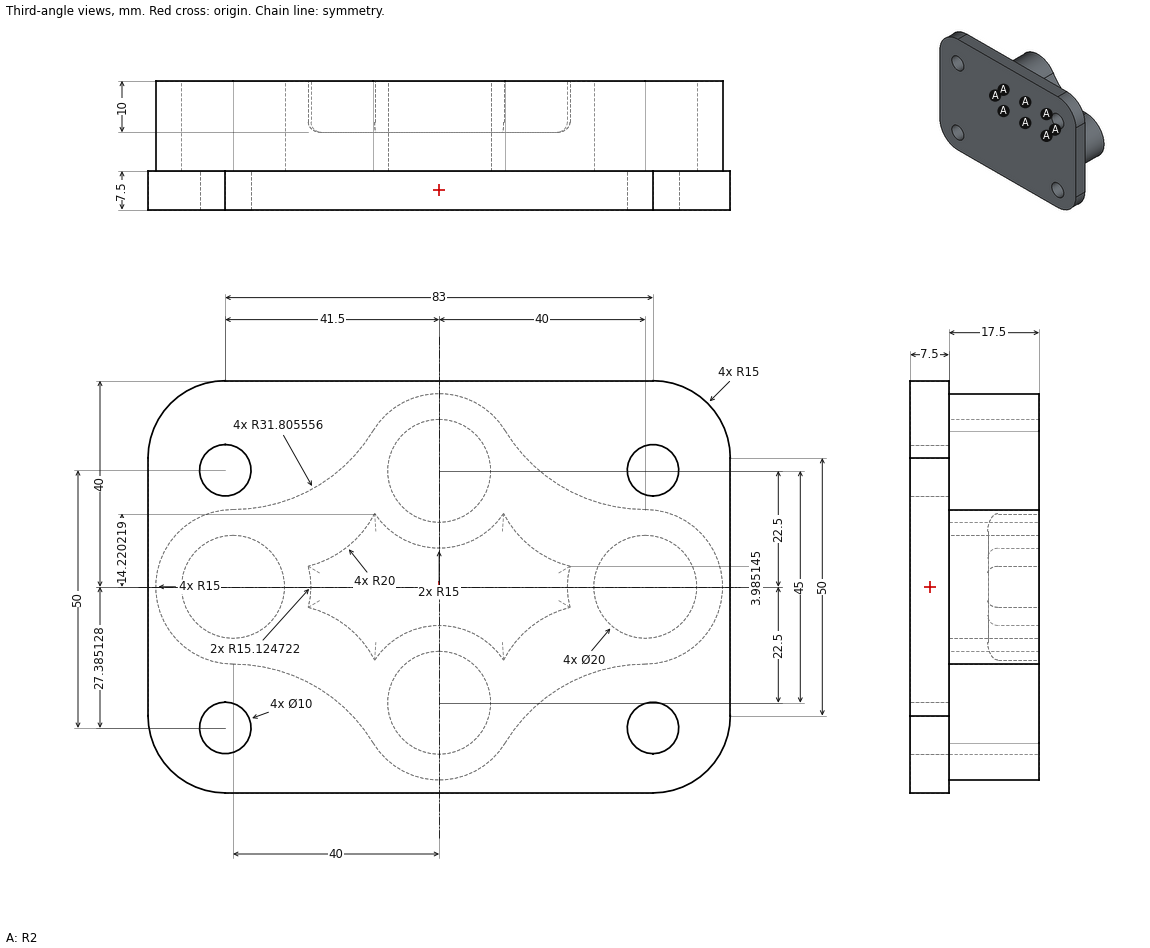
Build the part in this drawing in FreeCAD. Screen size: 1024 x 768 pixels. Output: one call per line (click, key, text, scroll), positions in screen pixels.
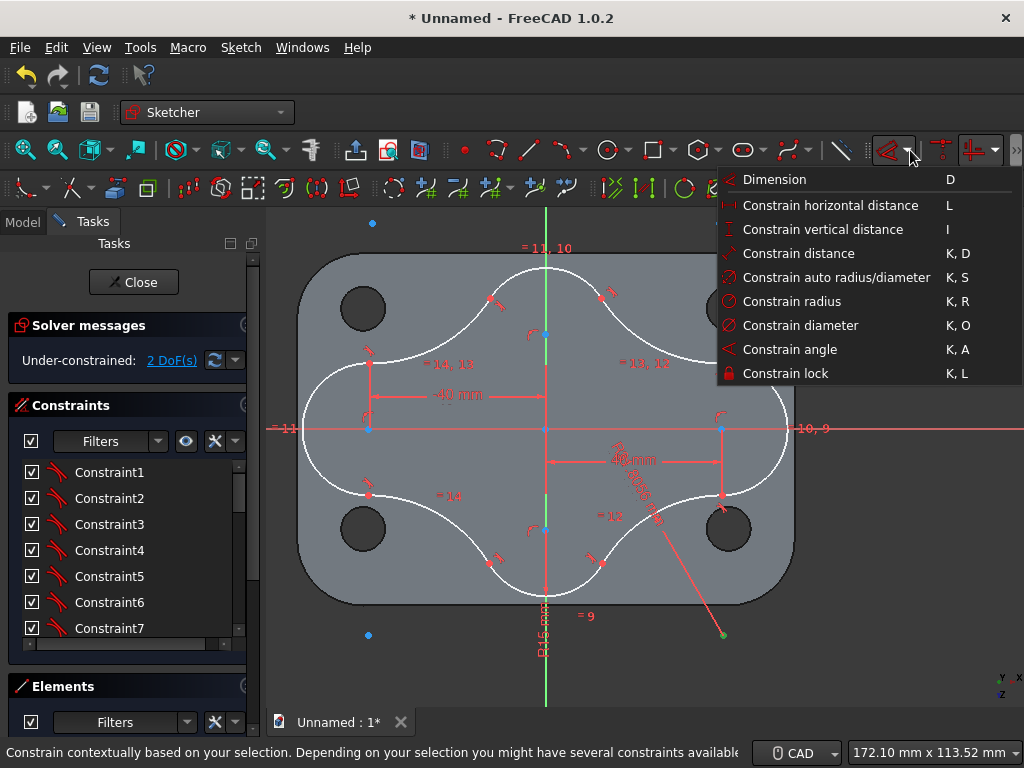
click(870, 205)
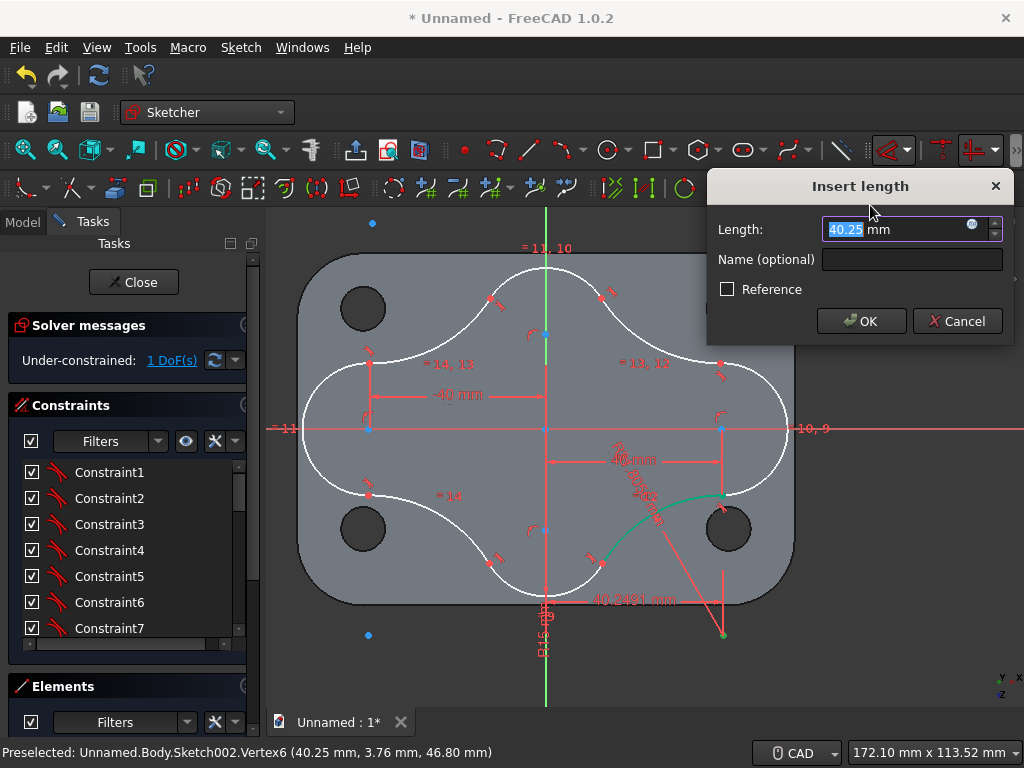
text(40)
key(Return)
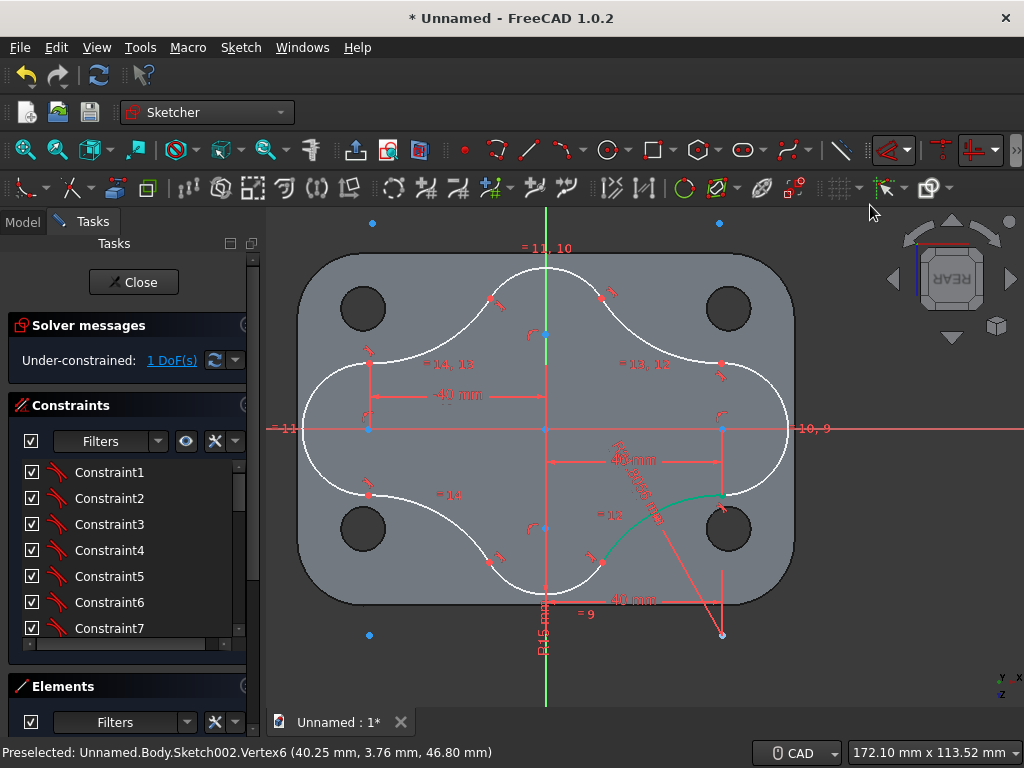
scroll(715, 582, down, 1)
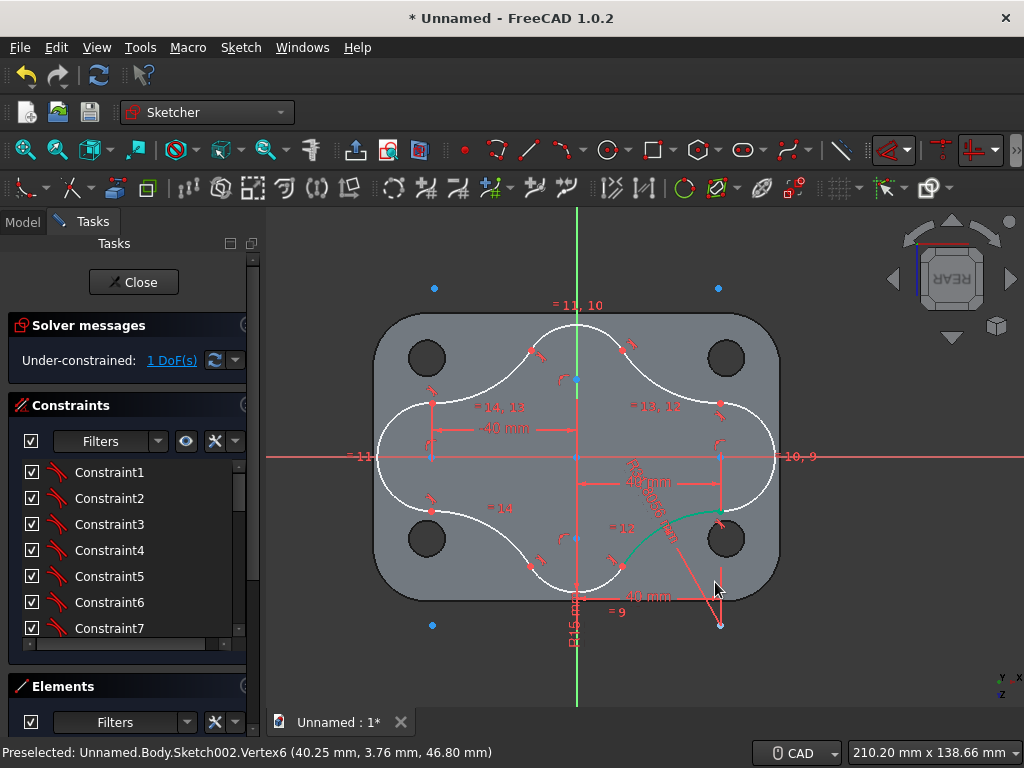
click(719, 288)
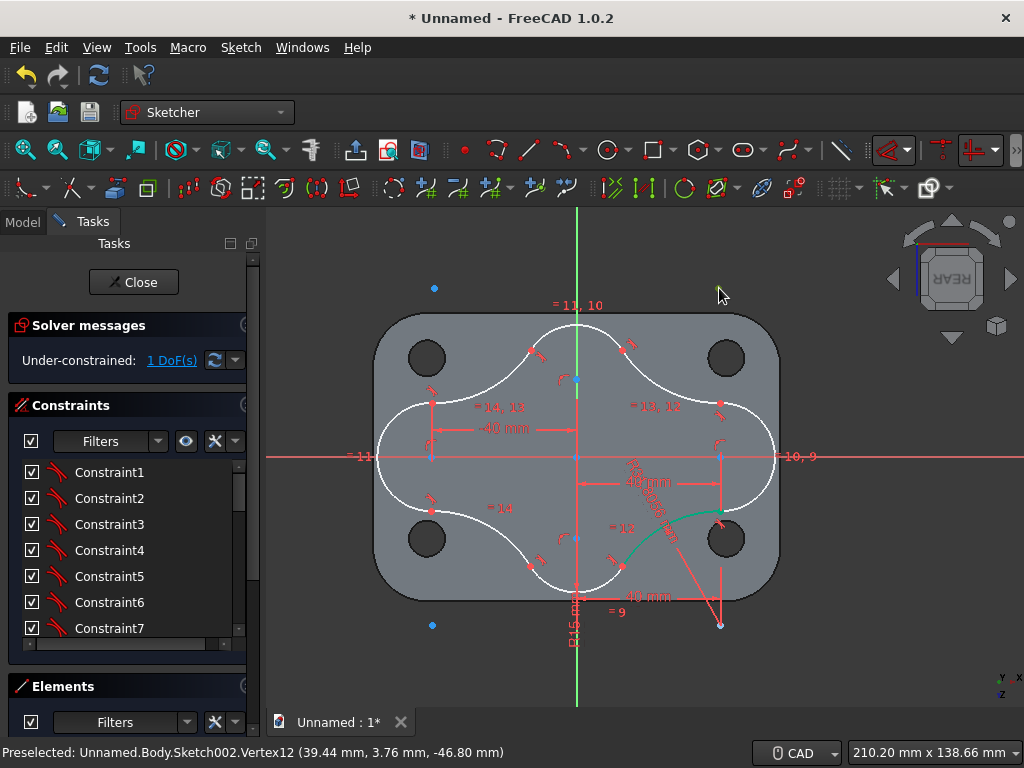
click(910, 150)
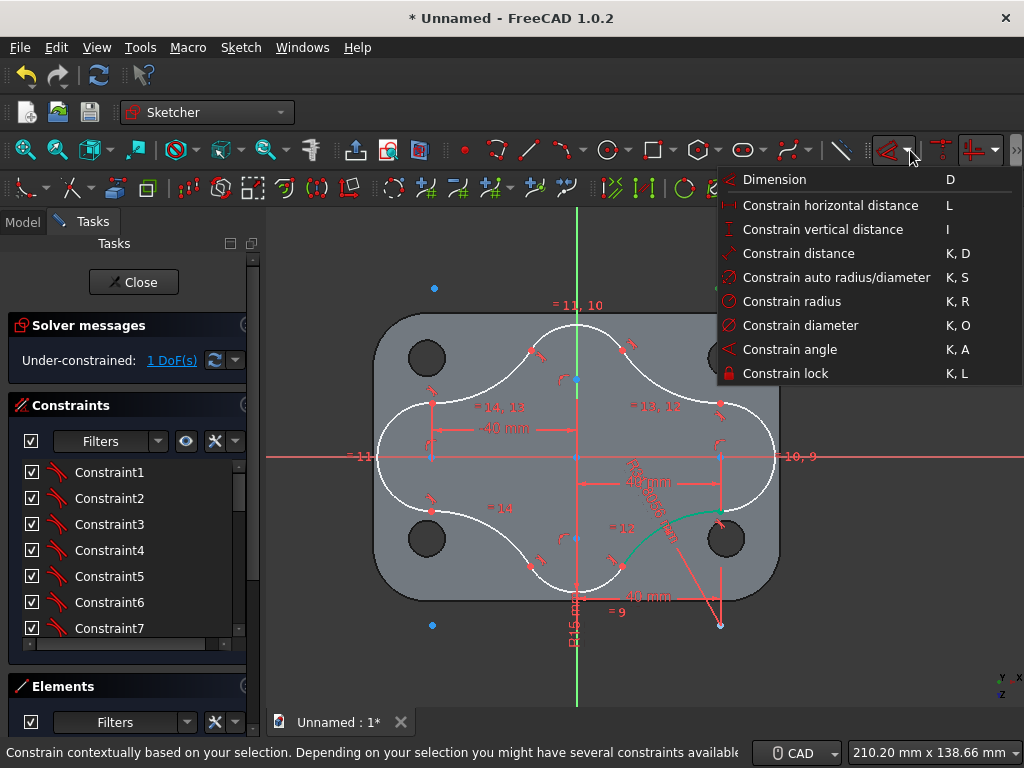
click(870, 205)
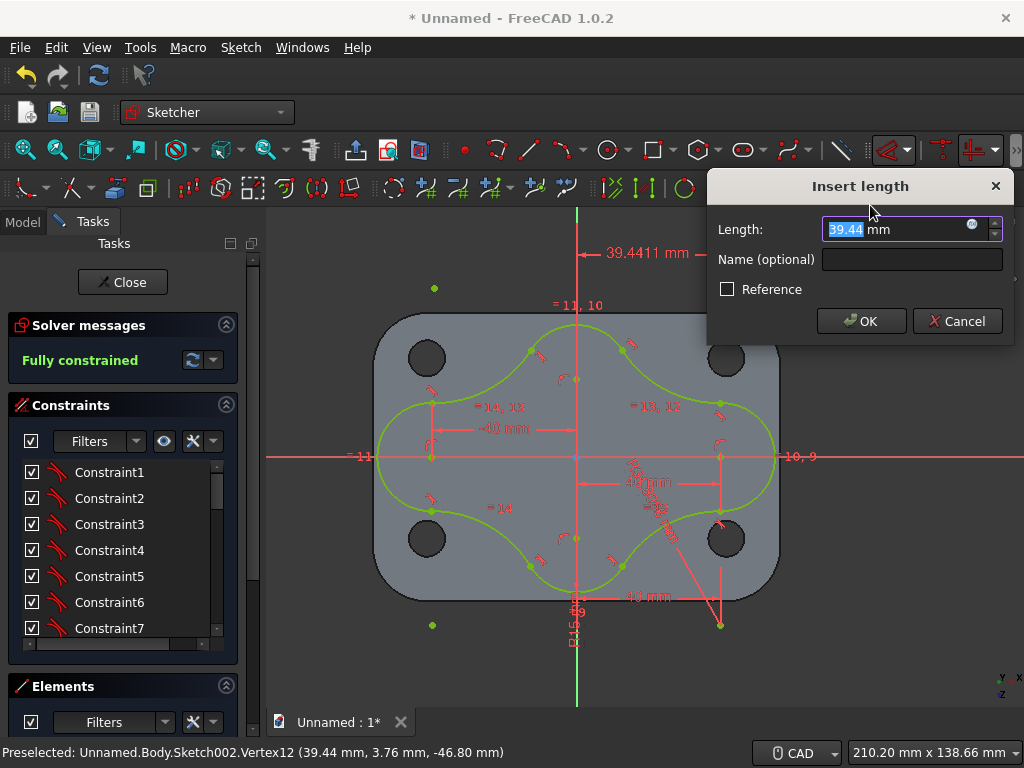
text(40)
key(Return)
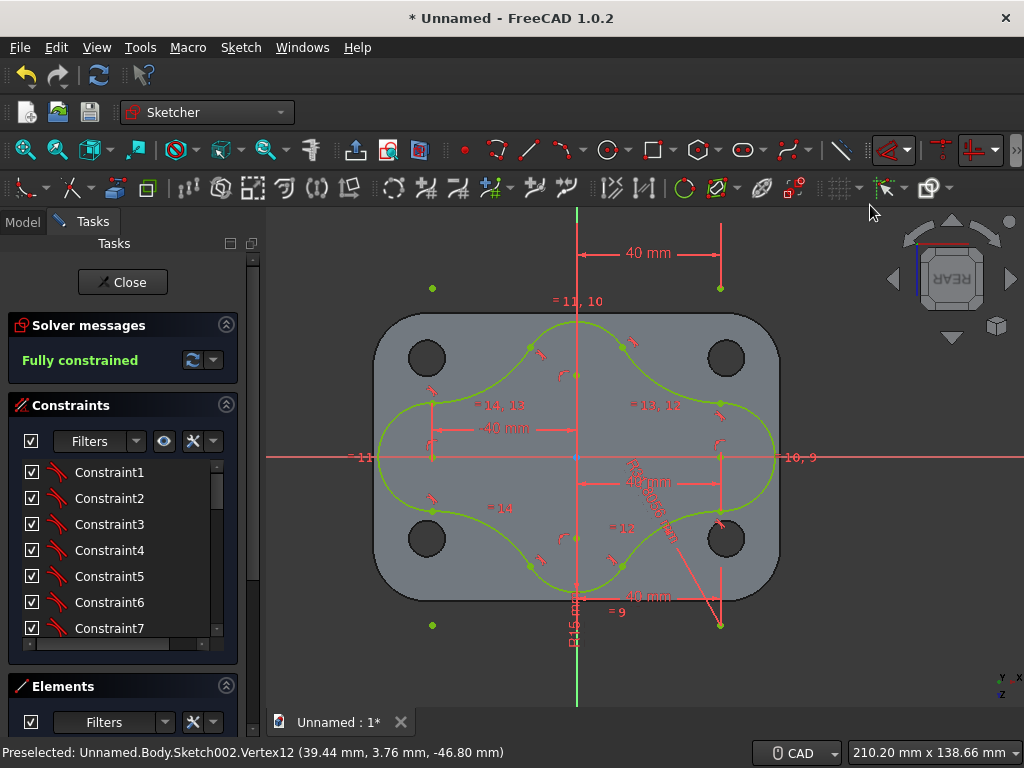
click(123, 282)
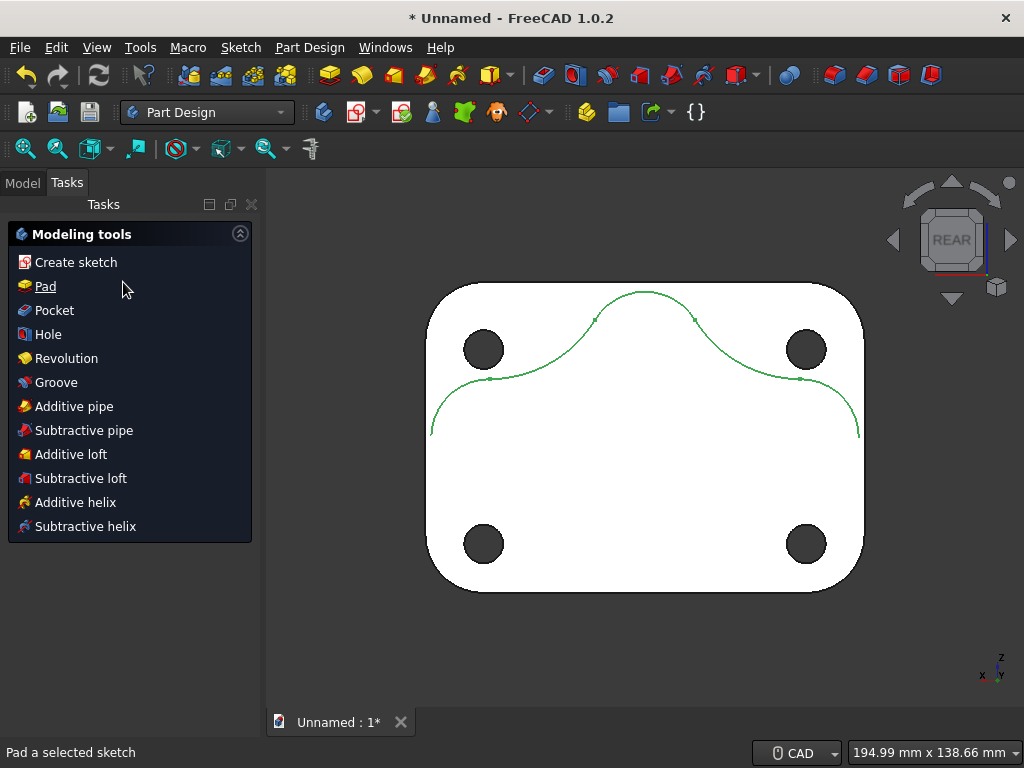
click(330, 76)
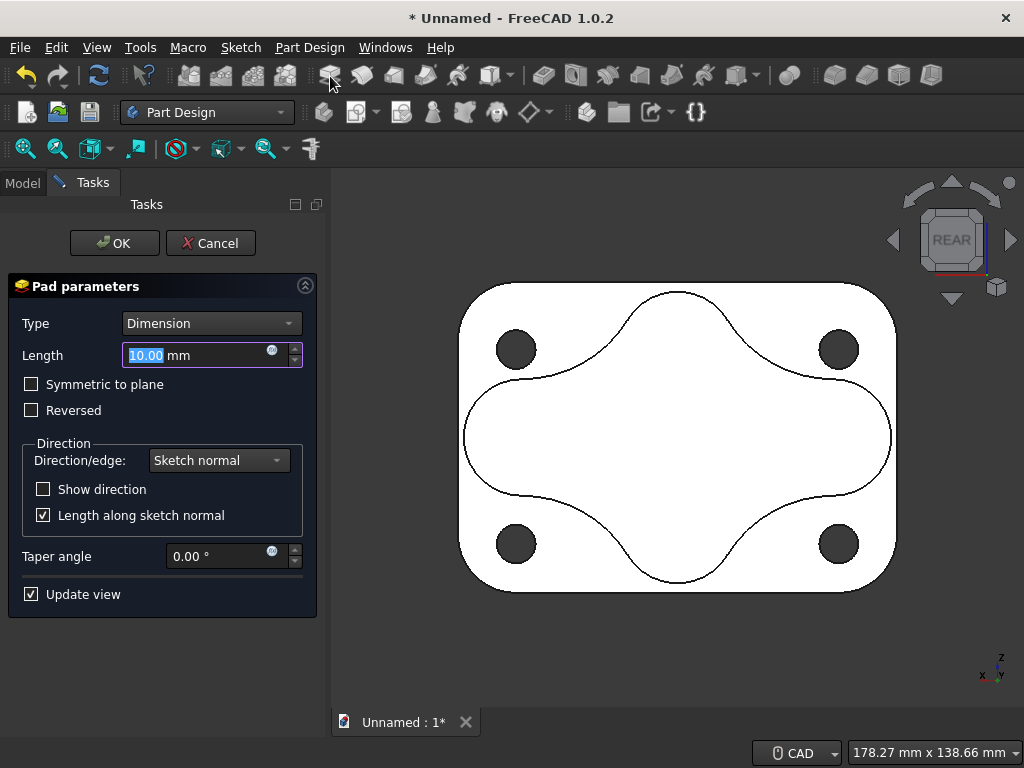
text(17.5)
key(Tab)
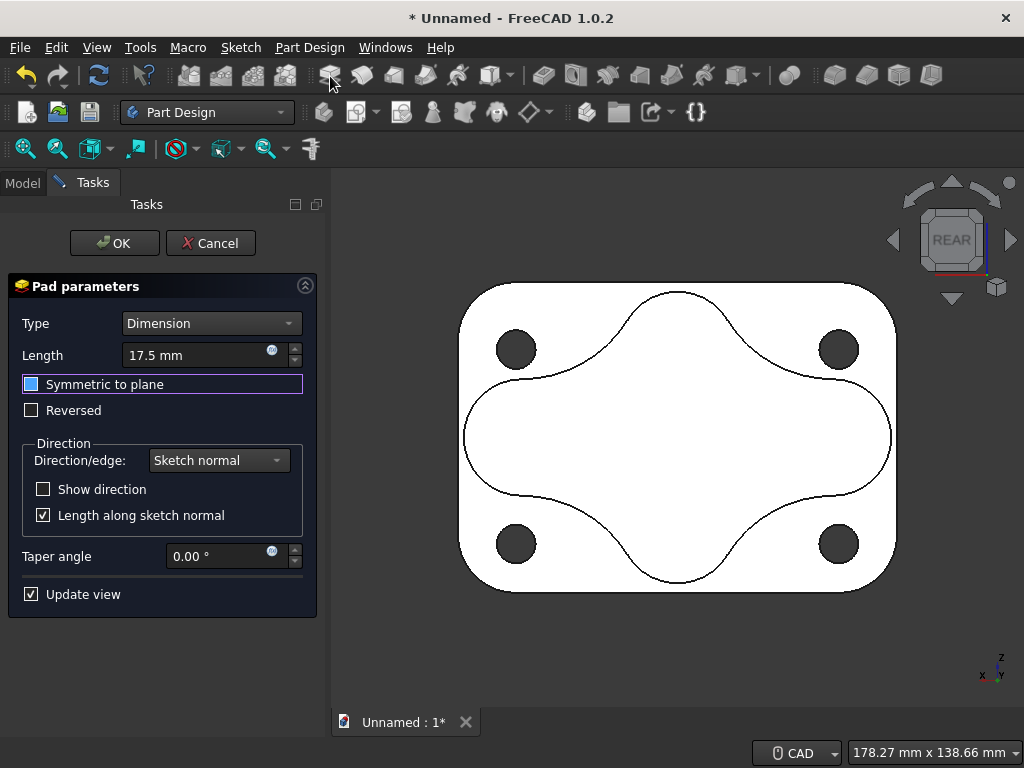
click(115, 243)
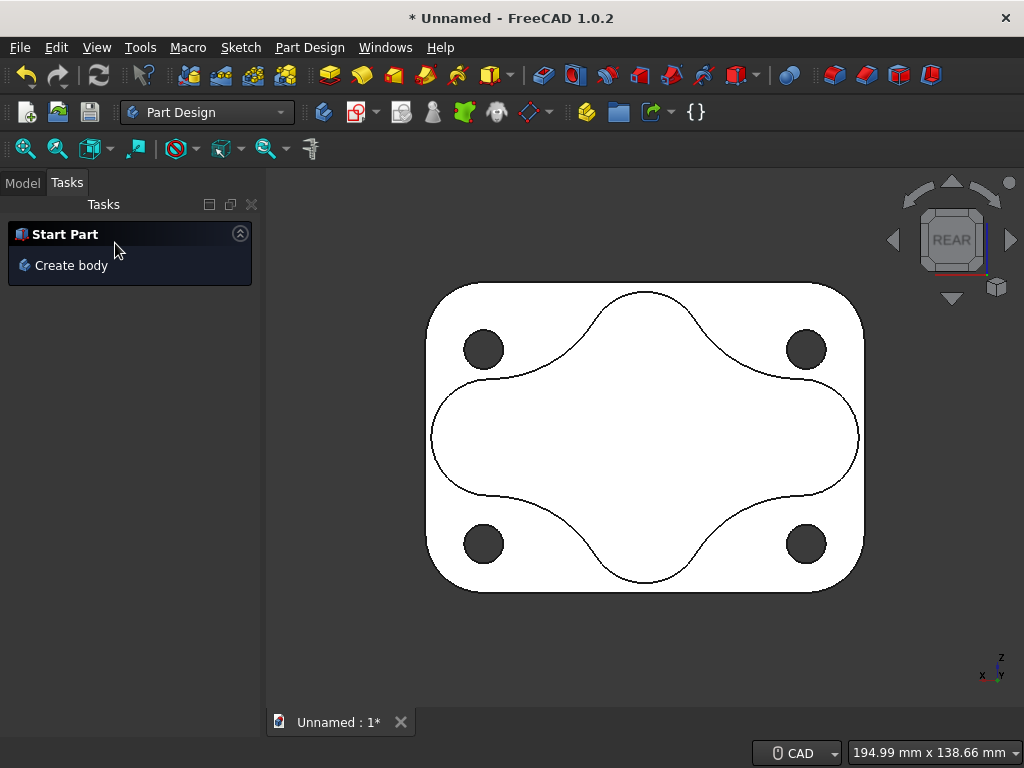
click(23, 182)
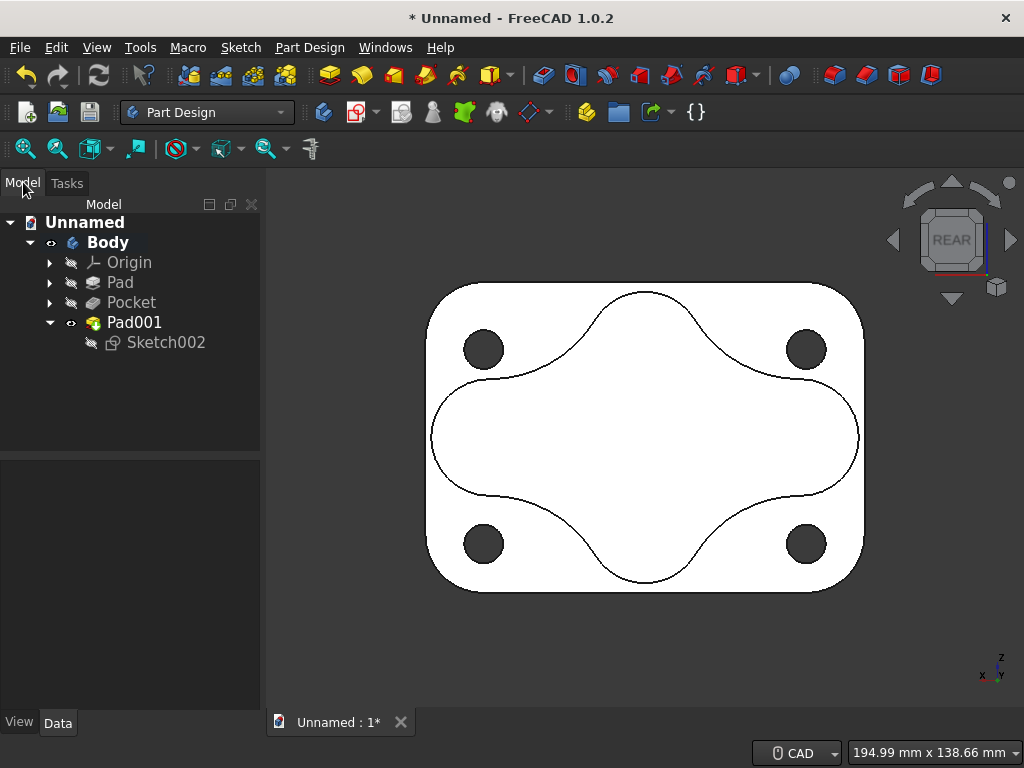
click(50, 263)